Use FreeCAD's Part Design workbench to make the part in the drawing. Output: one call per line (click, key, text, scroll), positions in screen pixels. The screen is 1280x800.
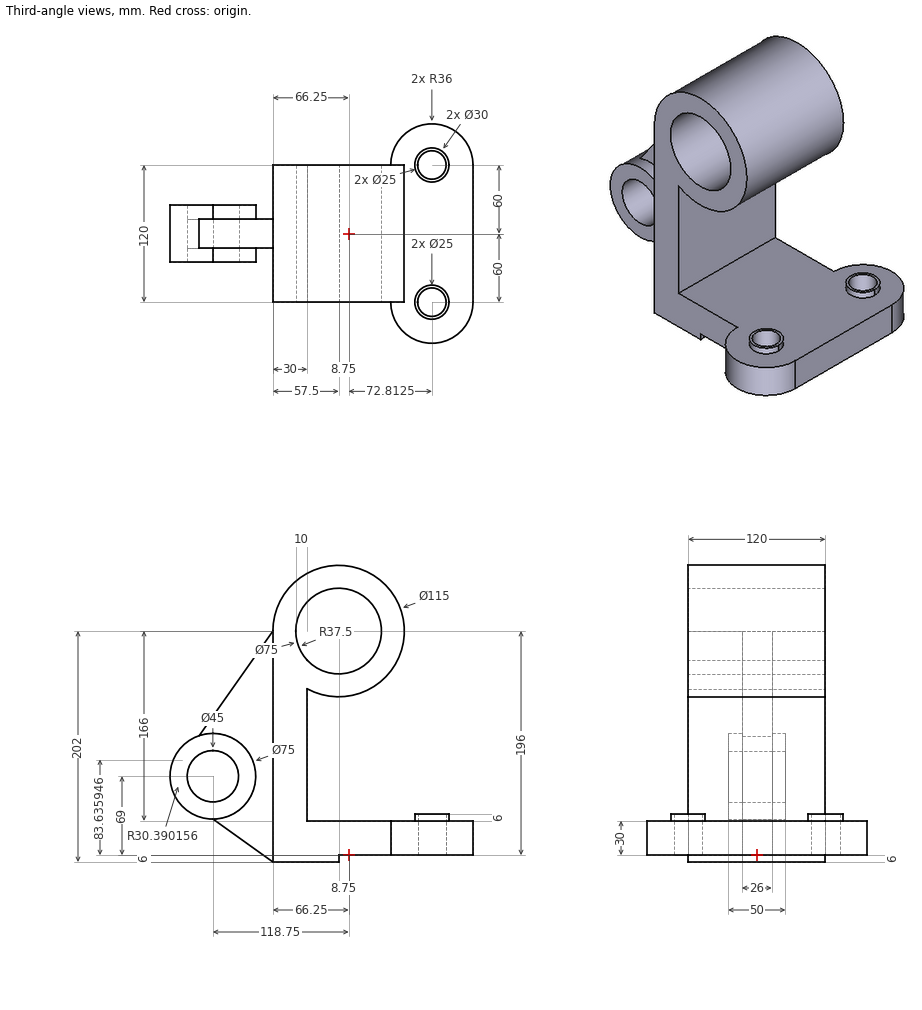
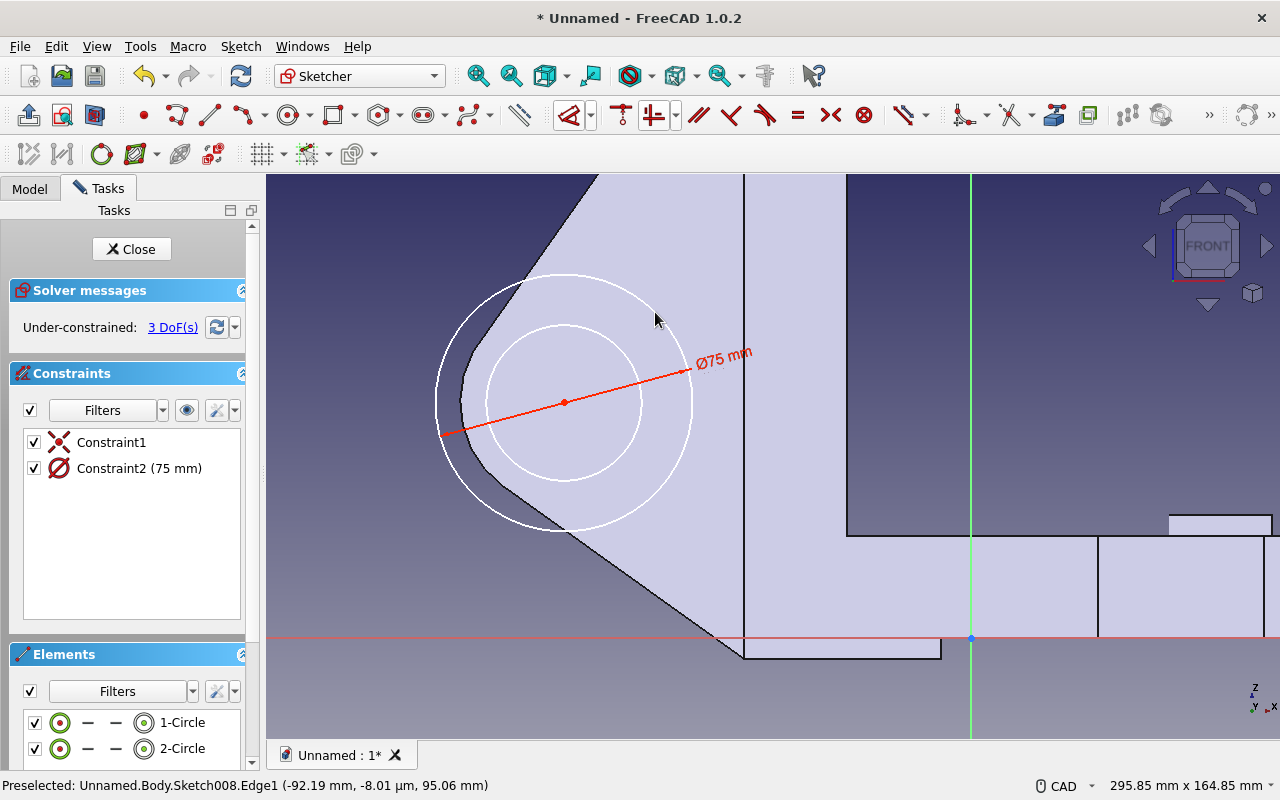
click(619, 348)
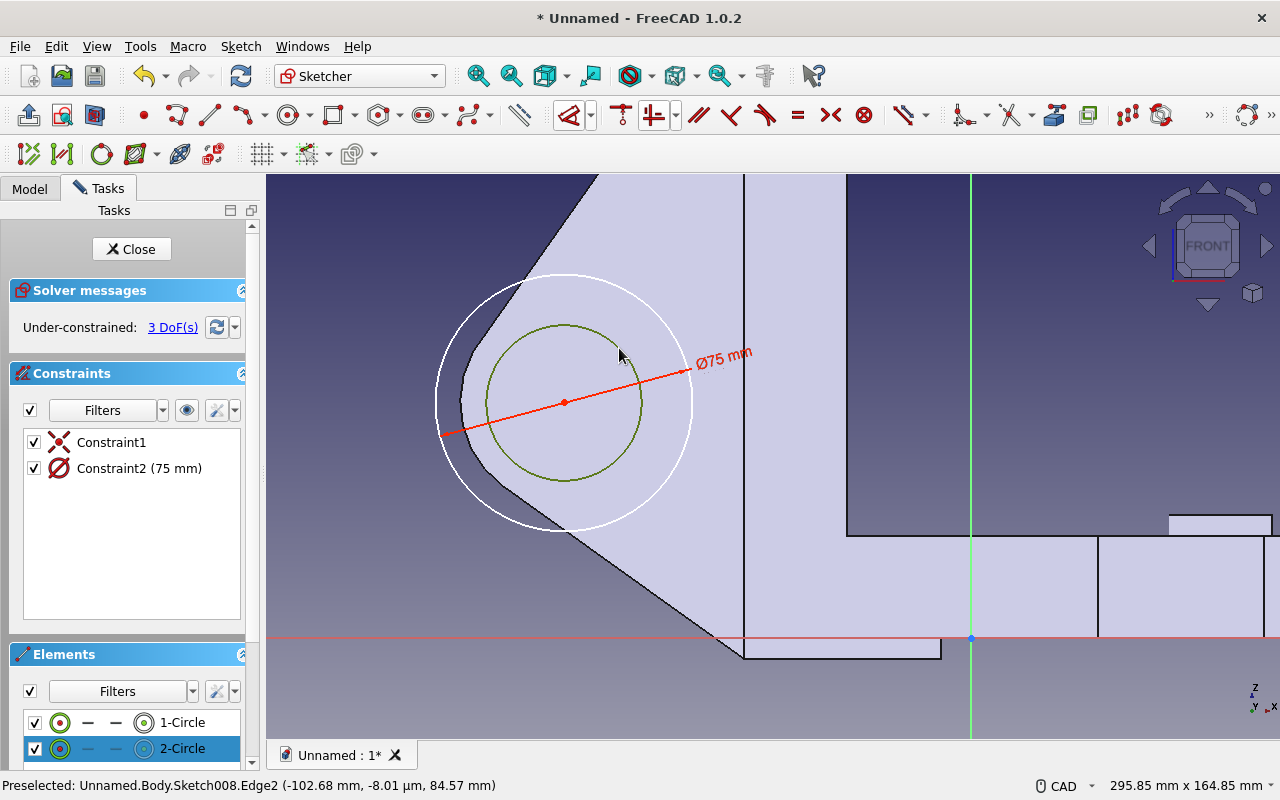
key(k)
key(o)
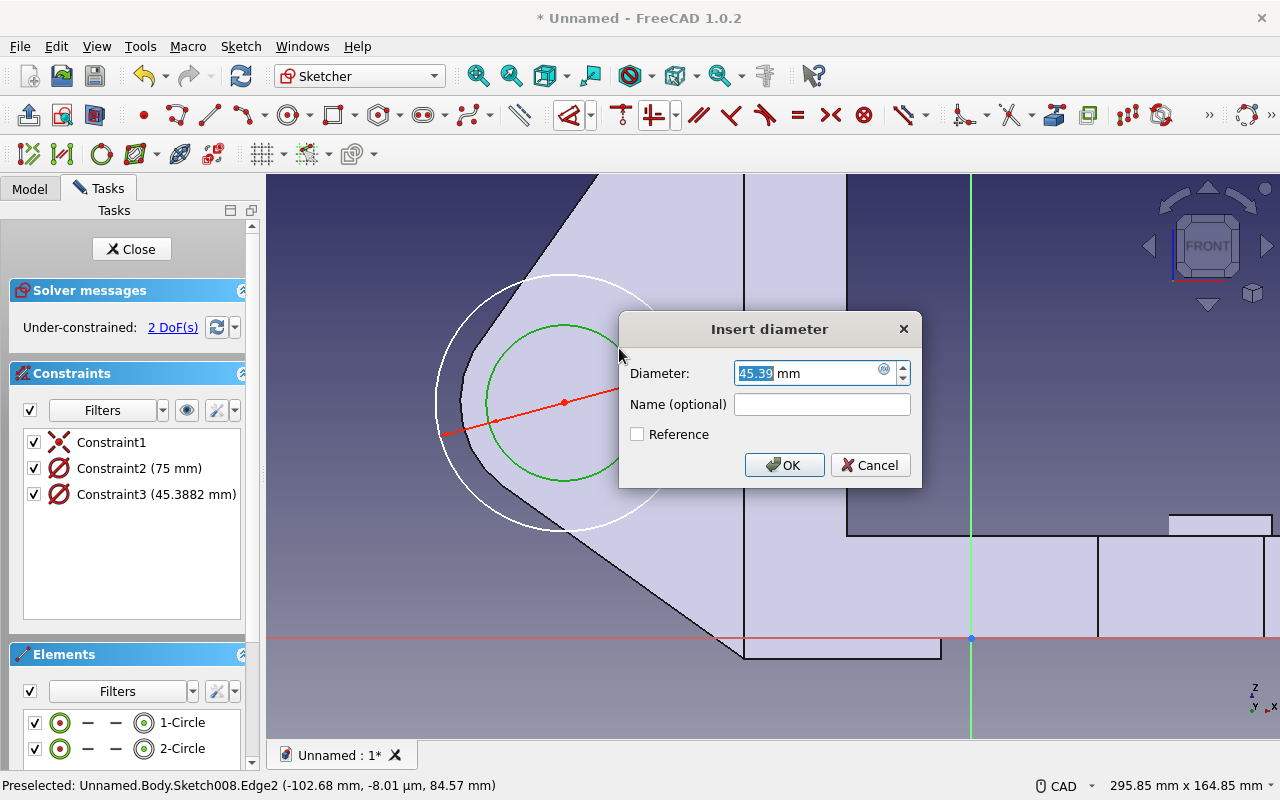
text(45)
key(Return)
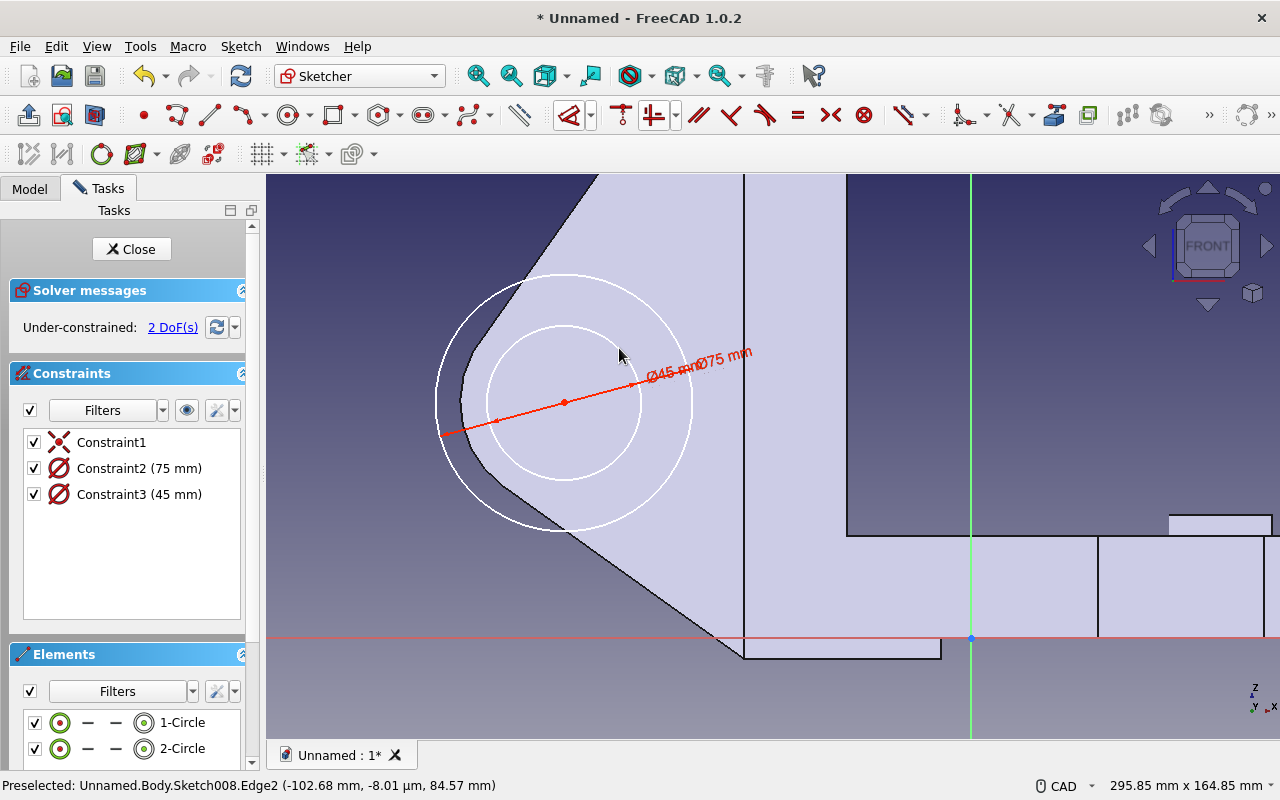
click(564, 403)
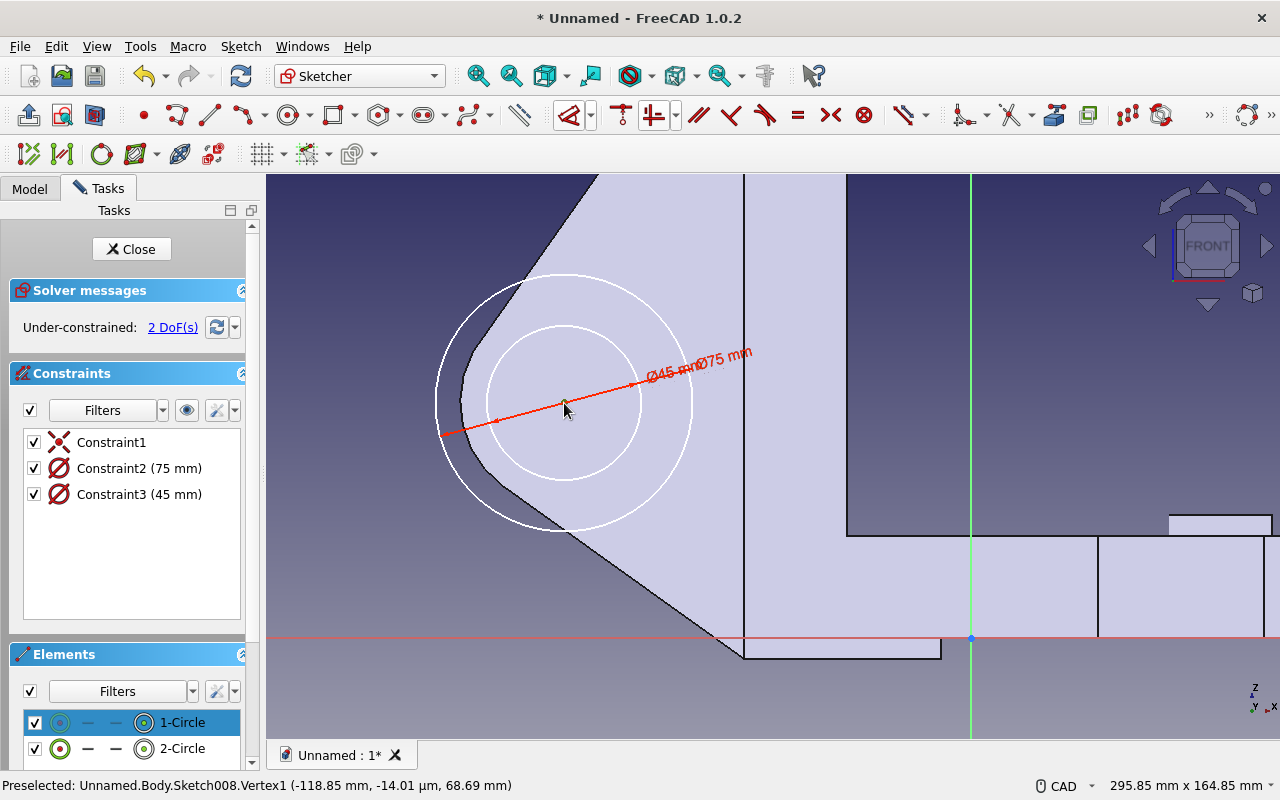
key(i)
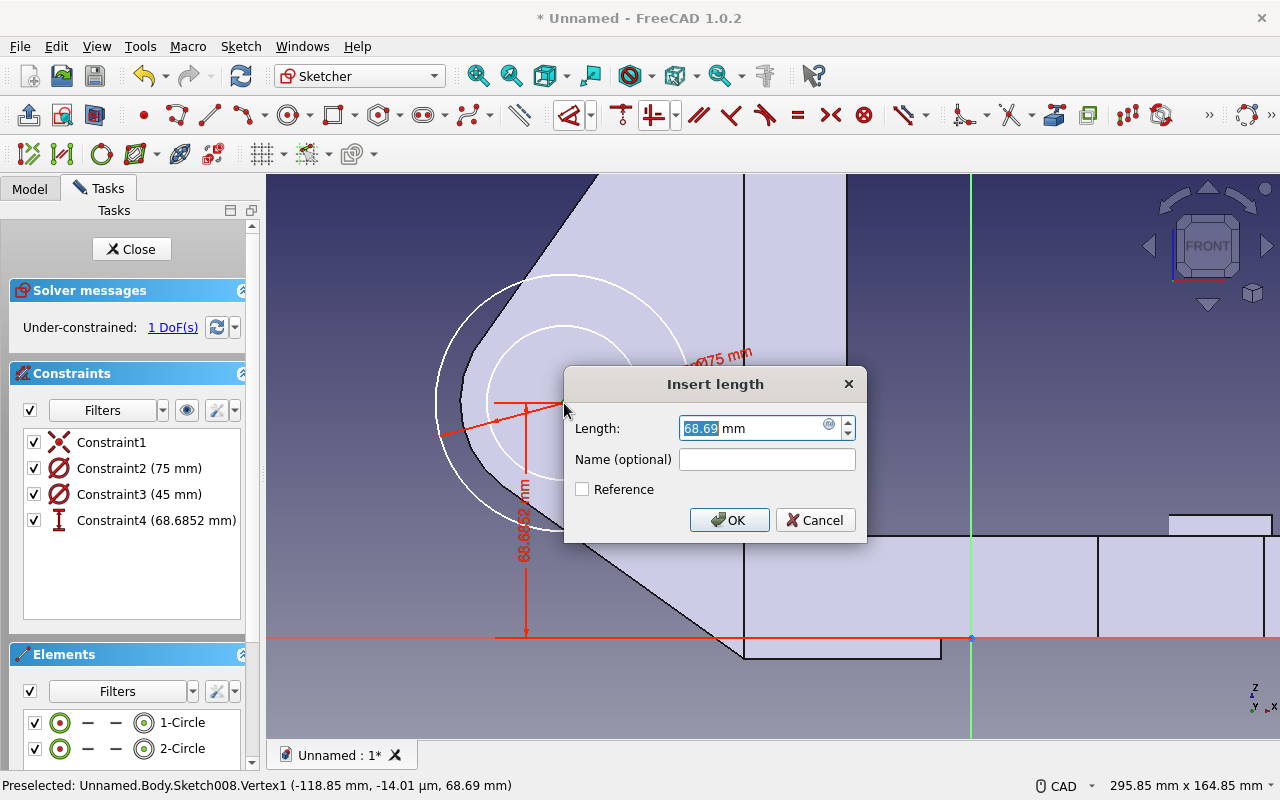
text(69)
key(Return)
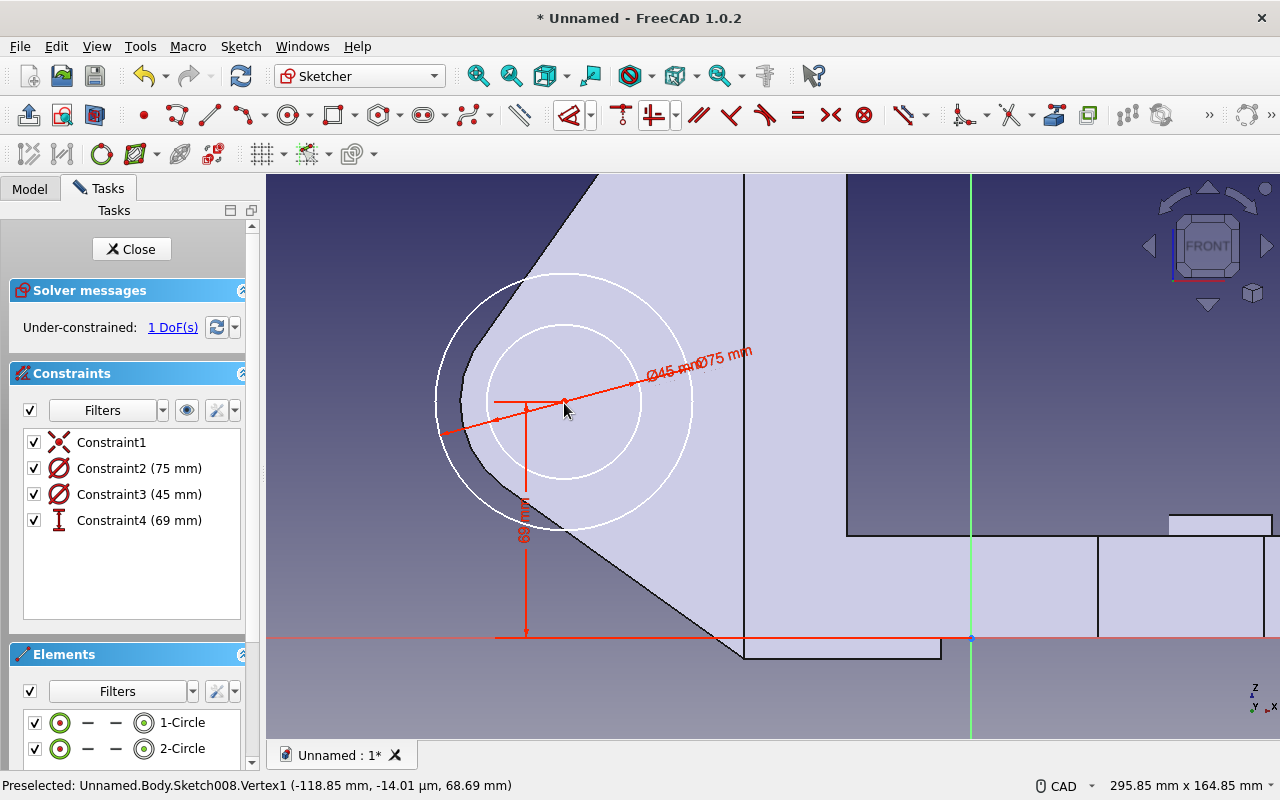
click(564, 402)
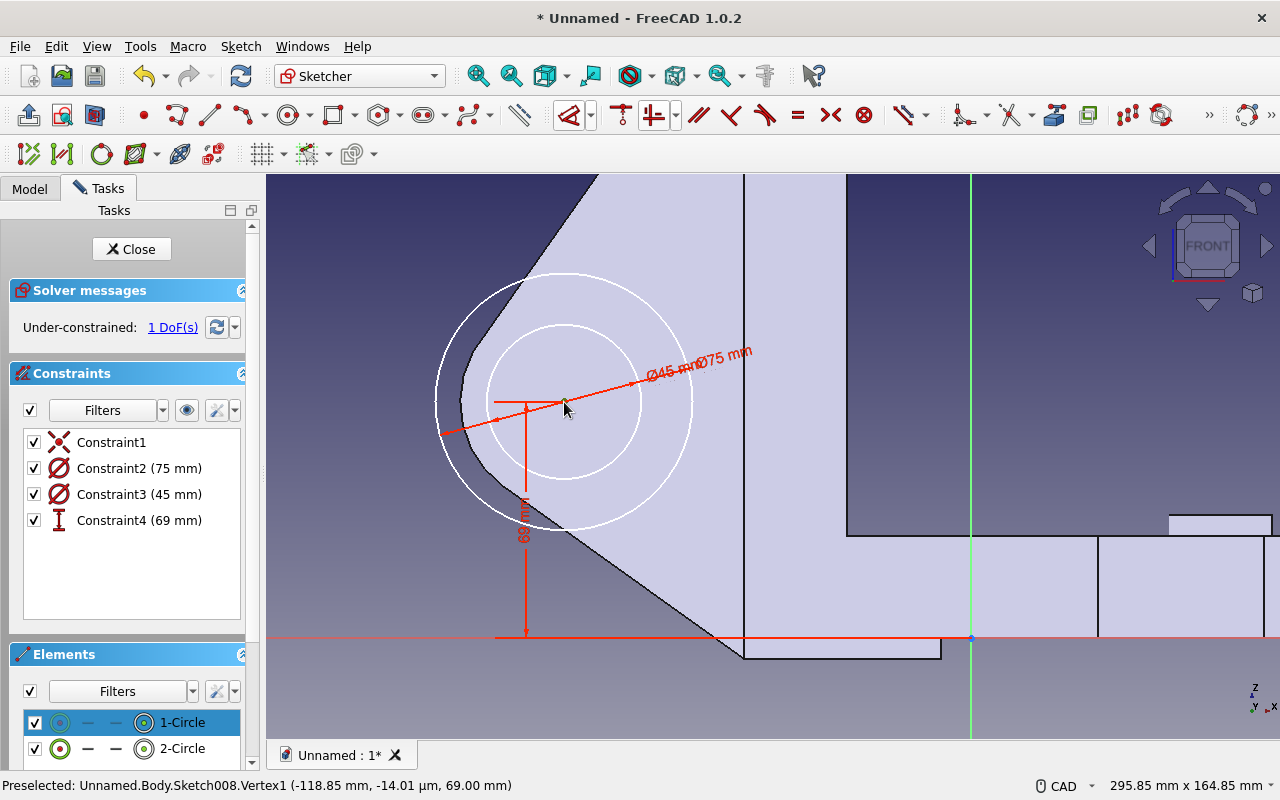
key(l)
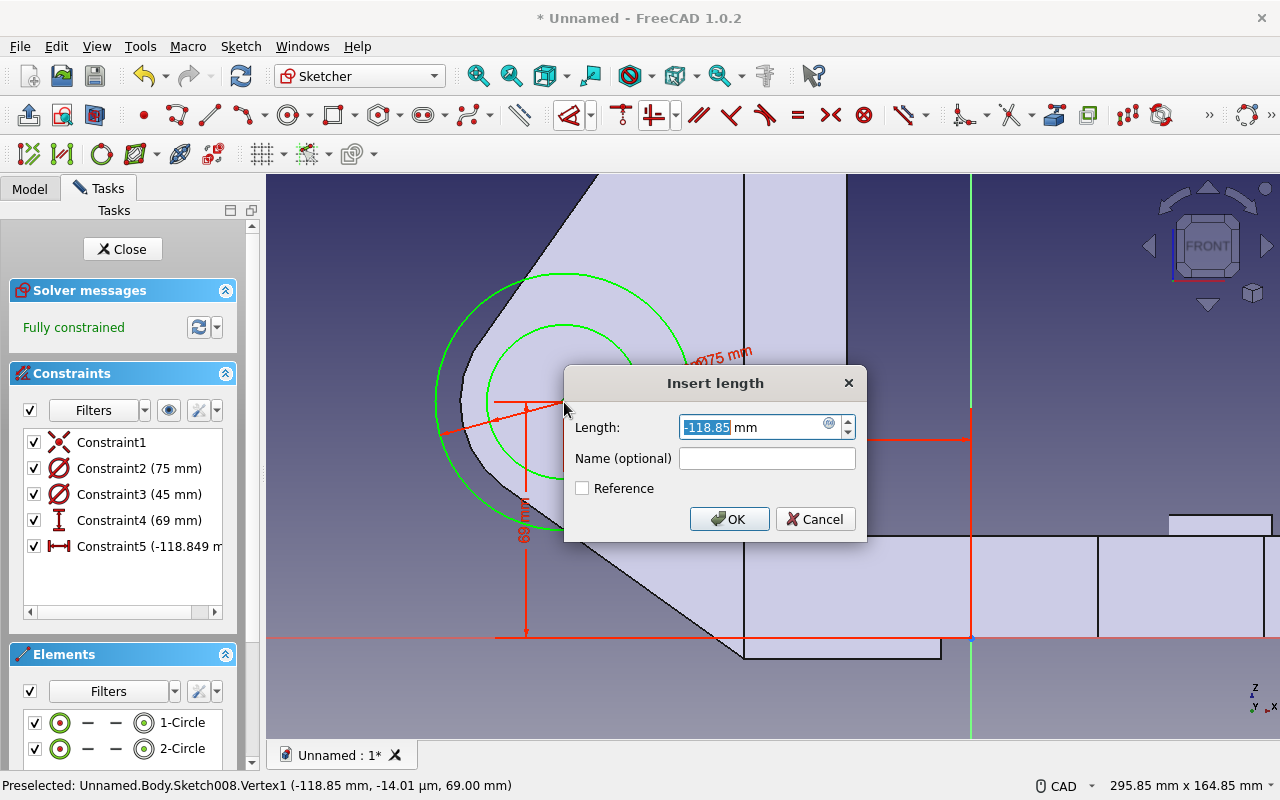
text(-118.75)
key(Return)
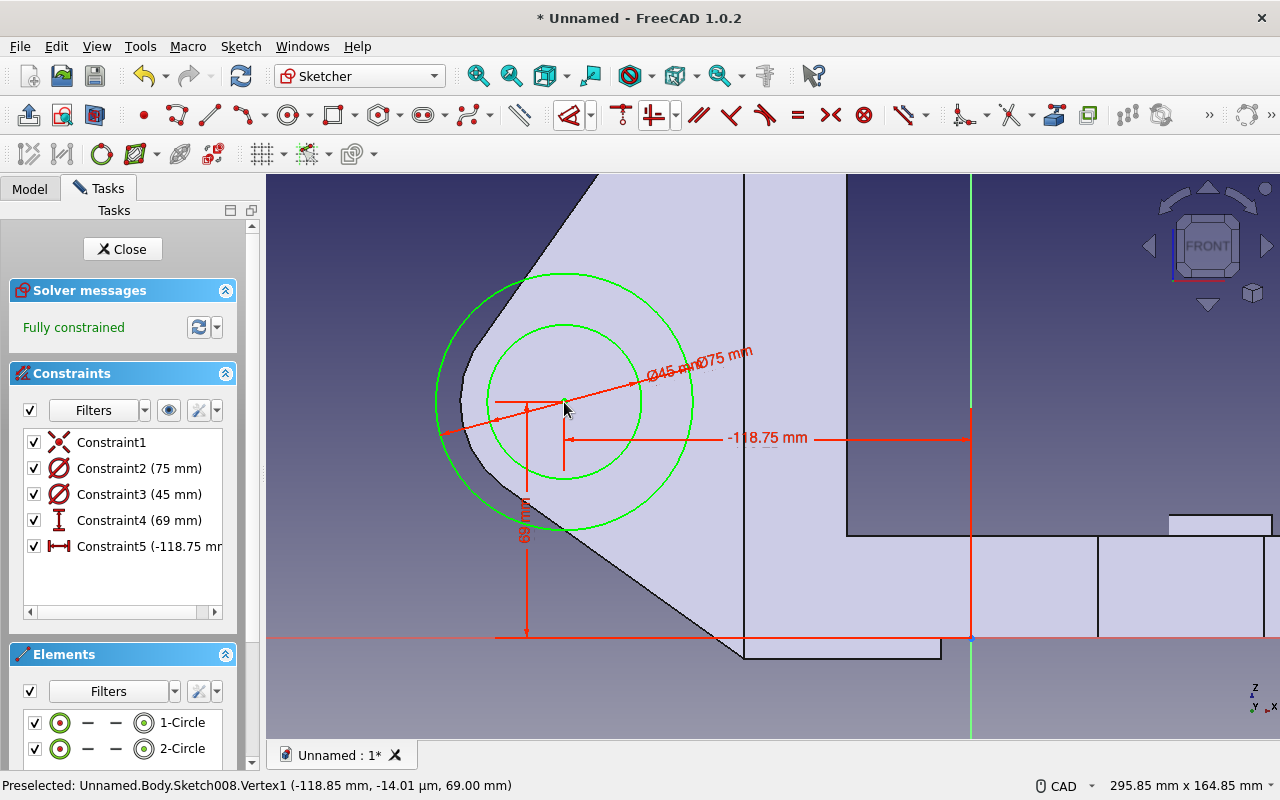
click(123, 249)